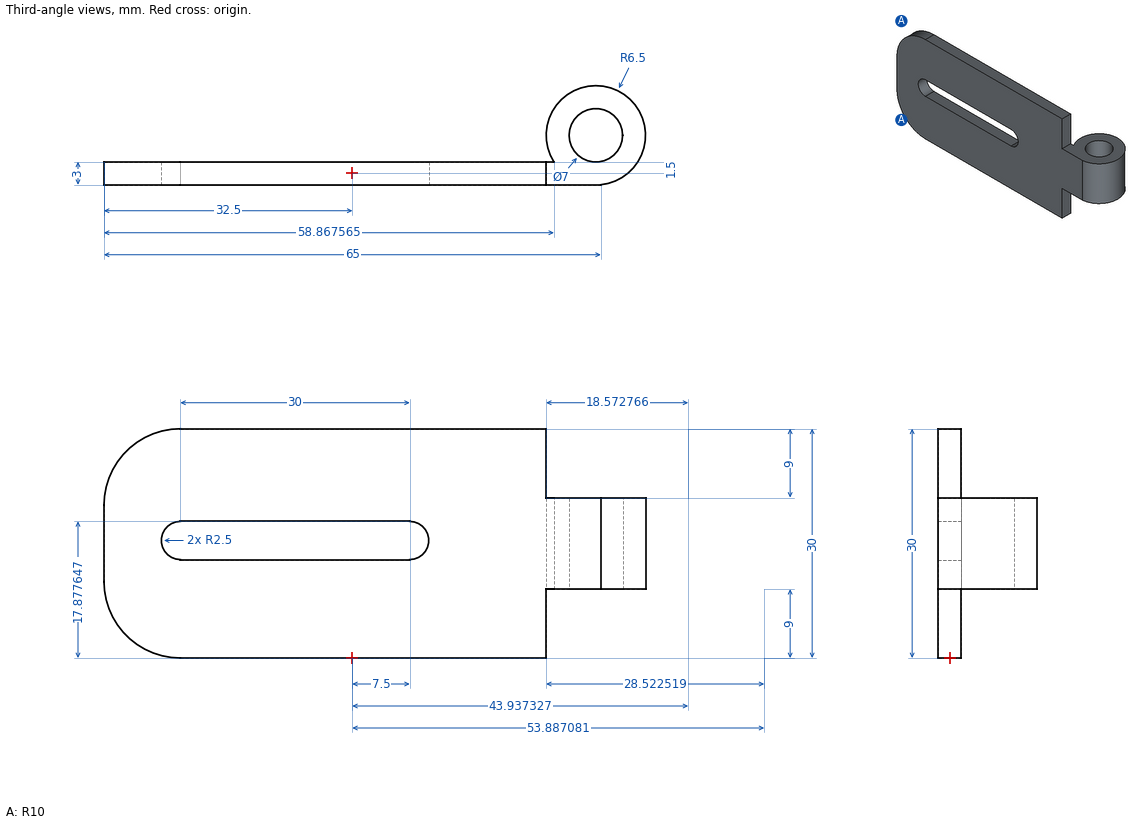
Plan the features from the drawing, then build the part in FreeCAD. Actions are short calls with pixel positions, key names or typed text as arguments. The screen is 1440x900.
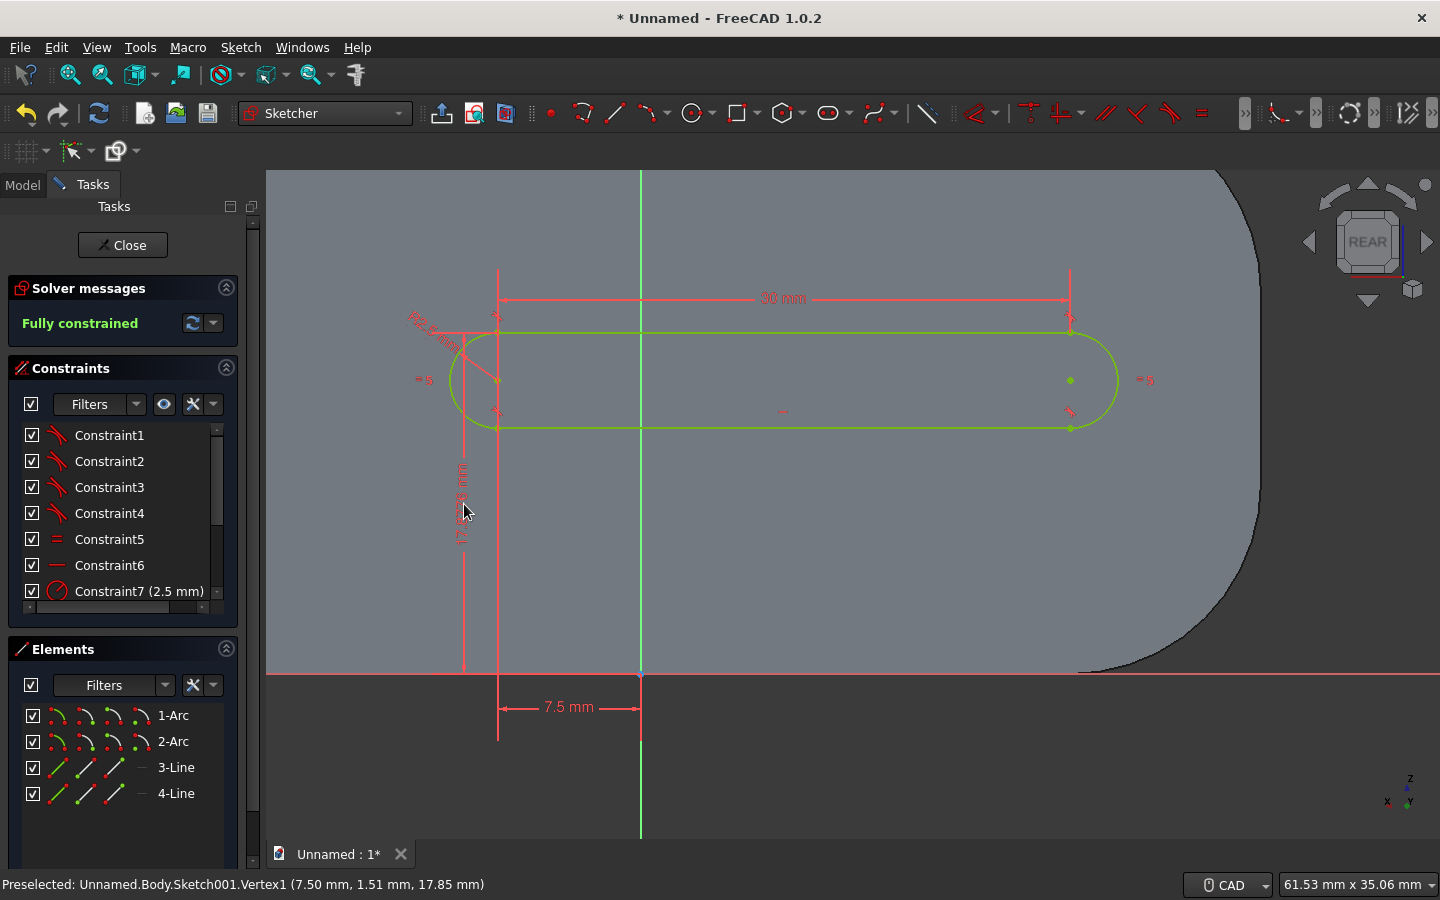
click(123, 245)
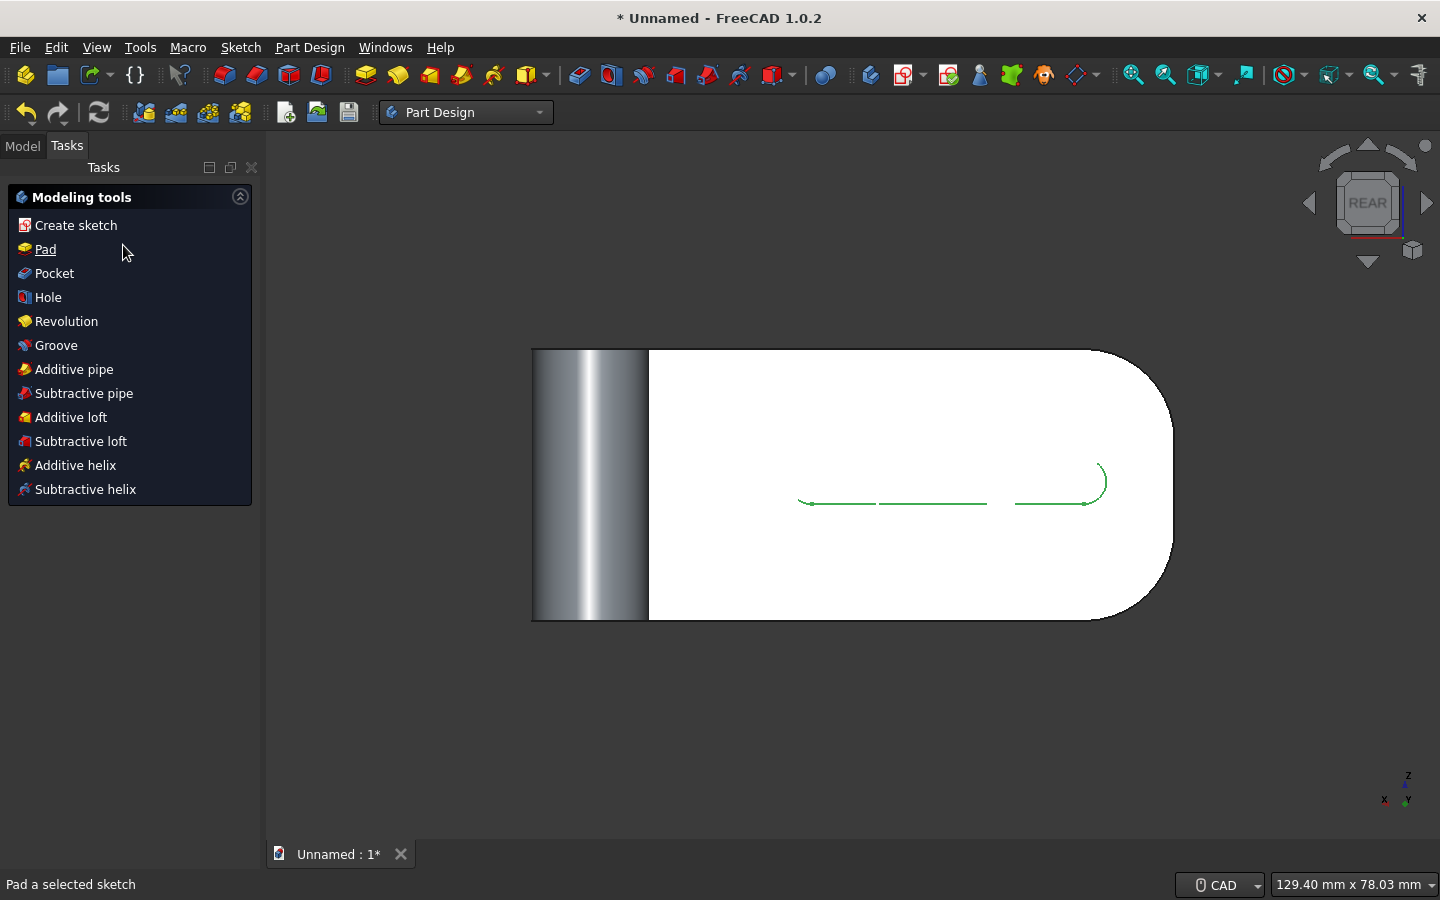
click(580, 76)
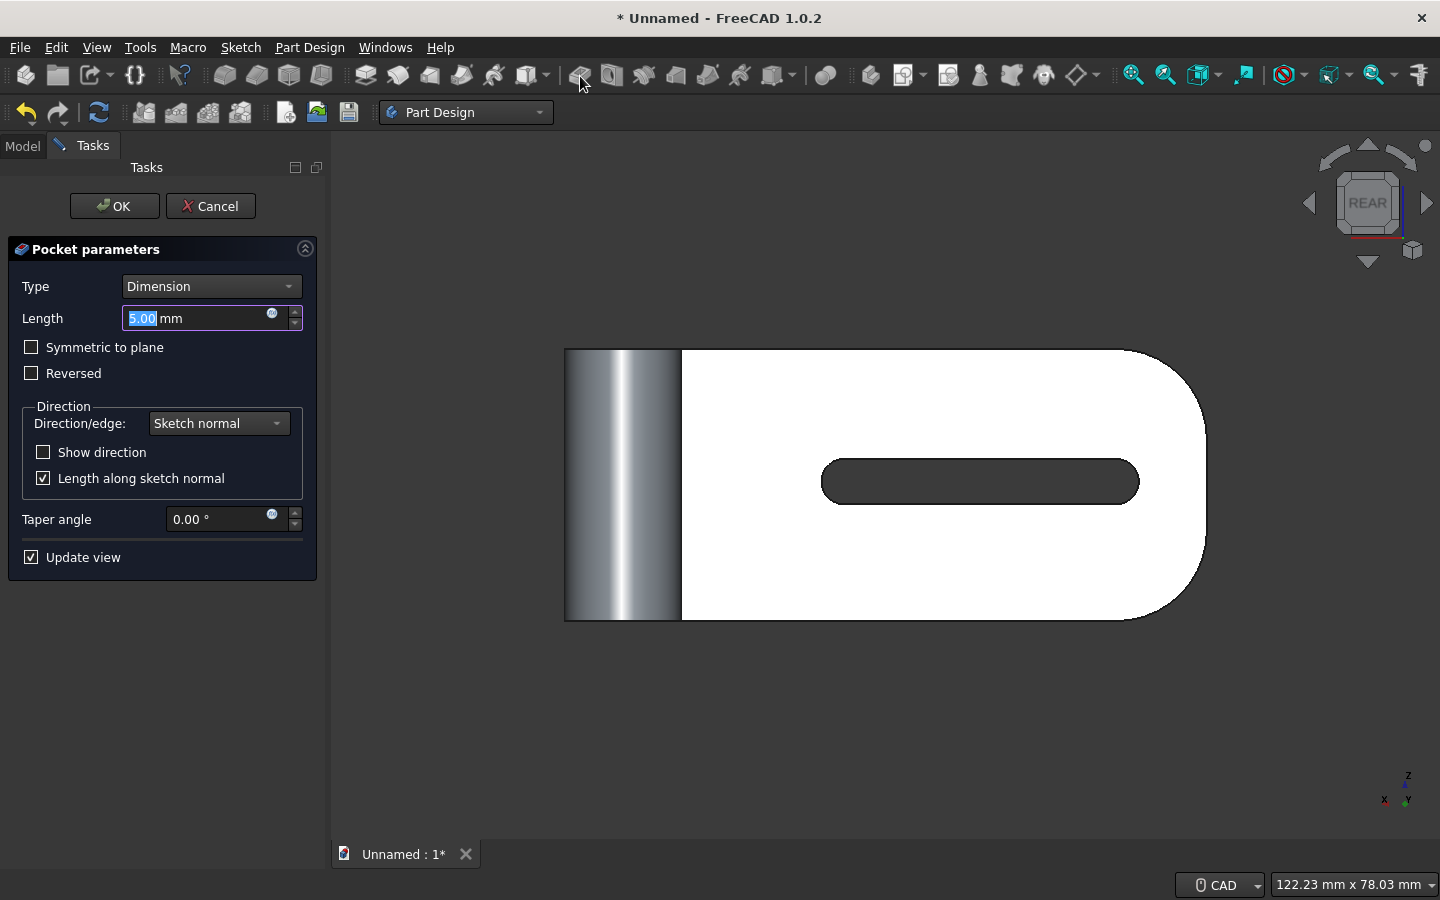
text(30)
key(Tab)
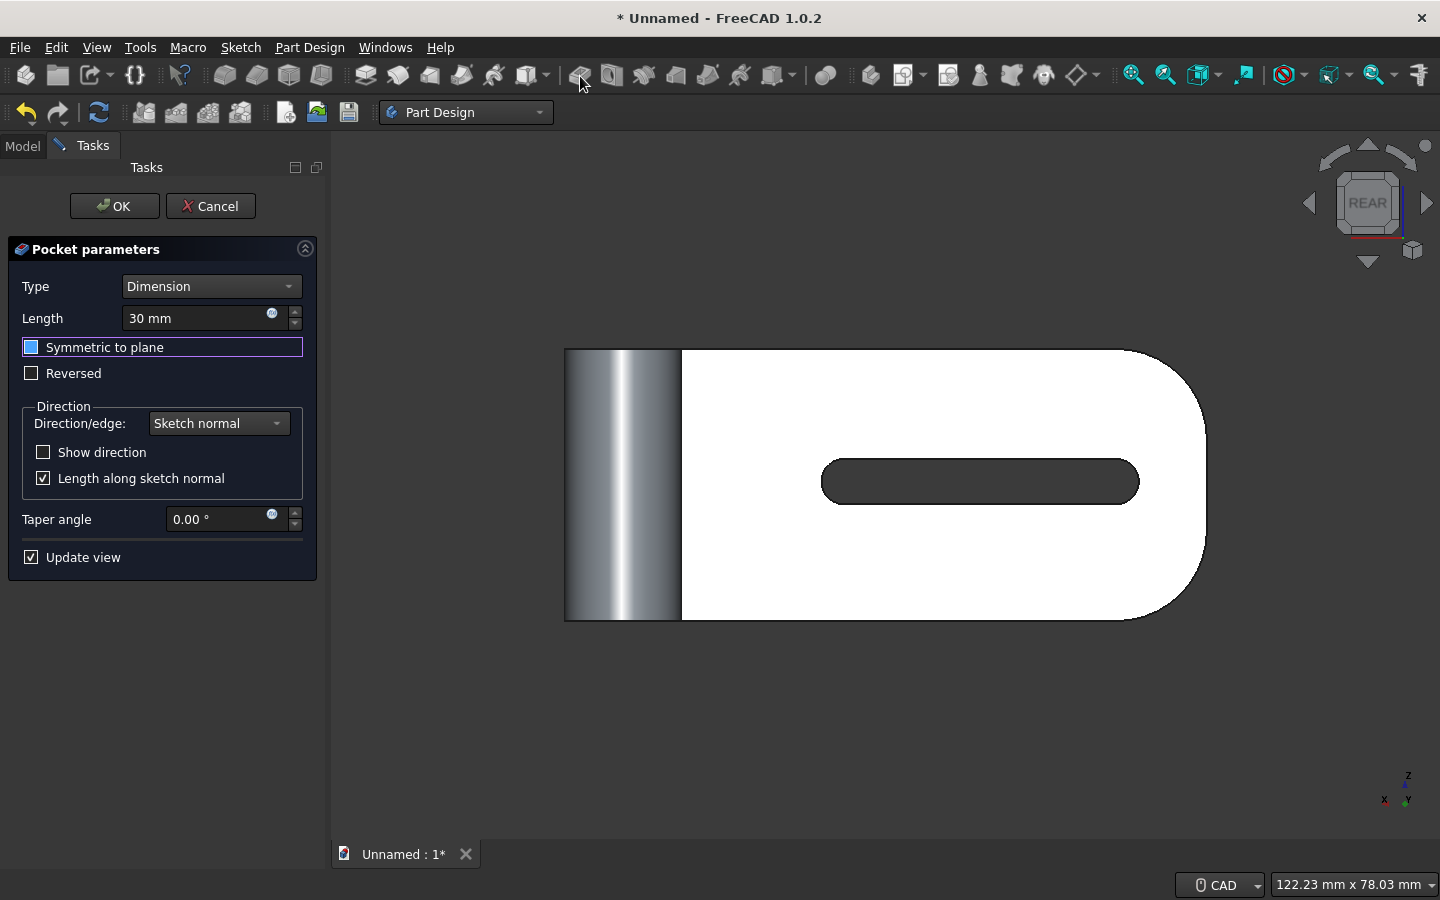
click(115, 206)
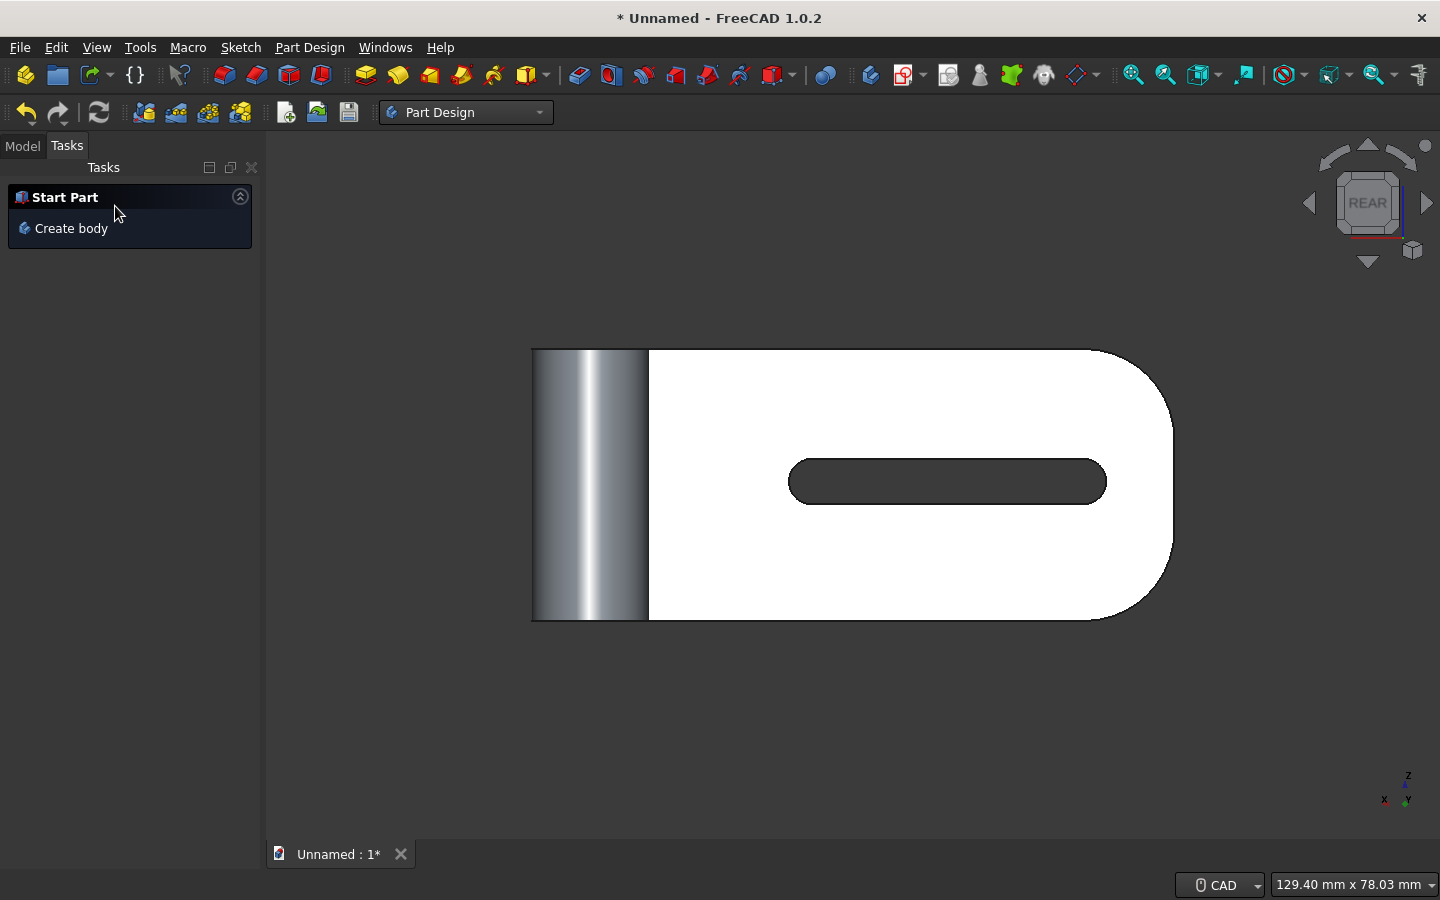
click(755, 406)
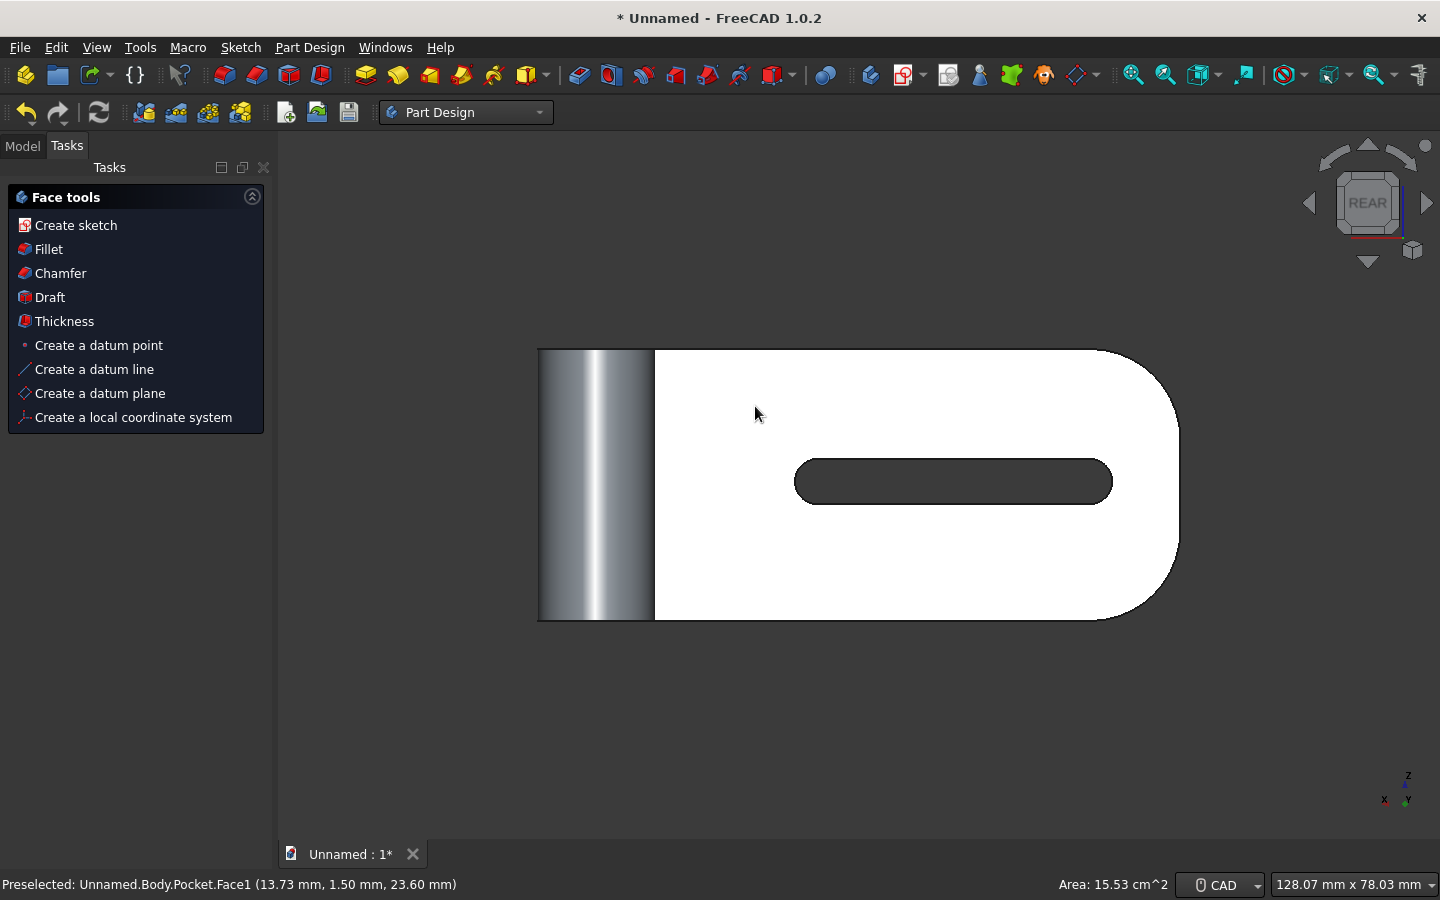
click(904, 76)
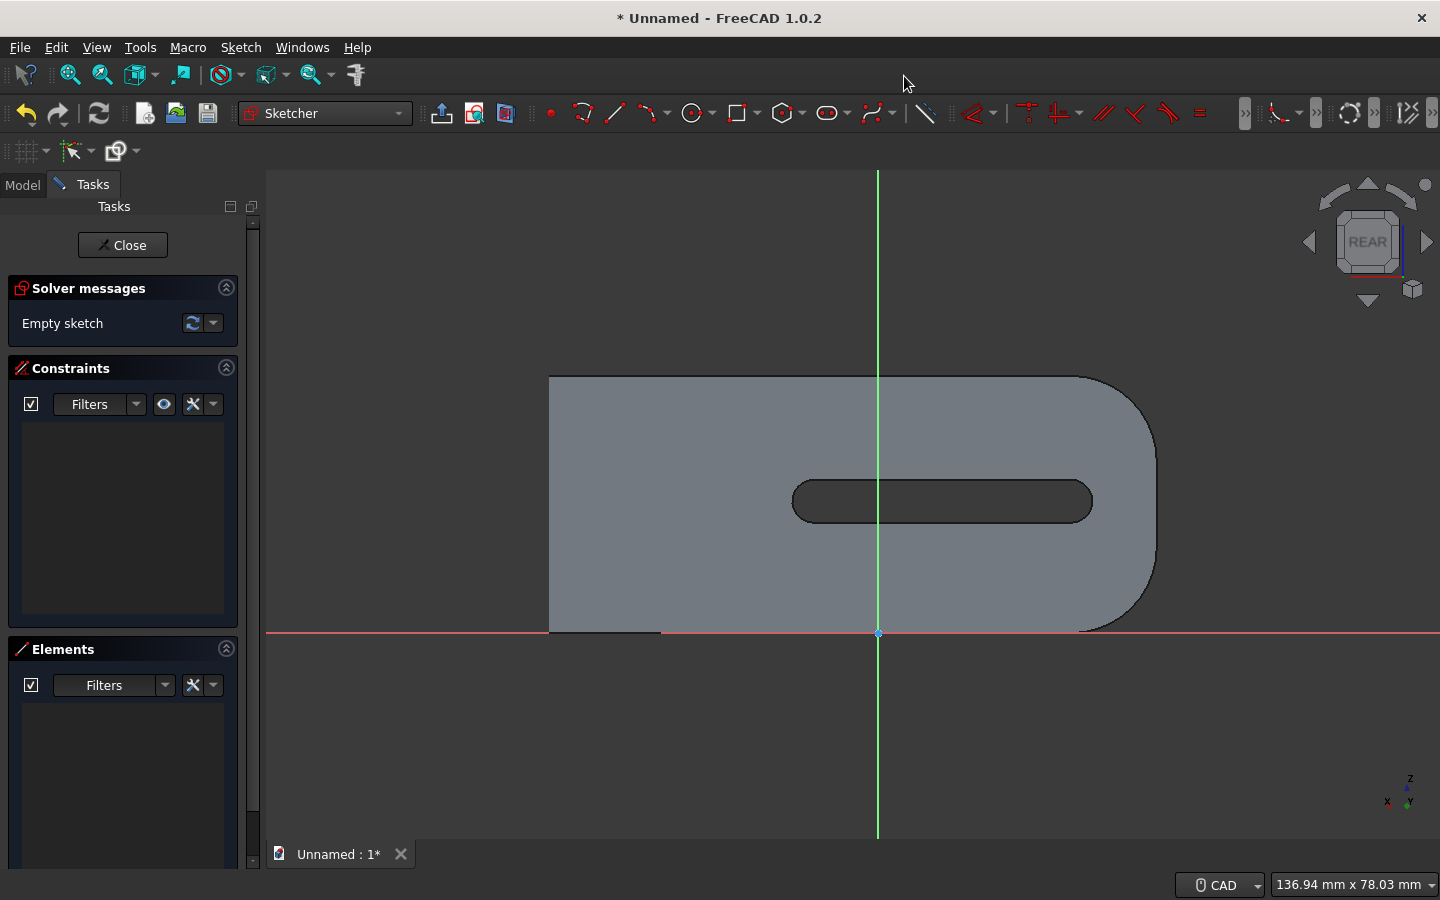
click(506, 114)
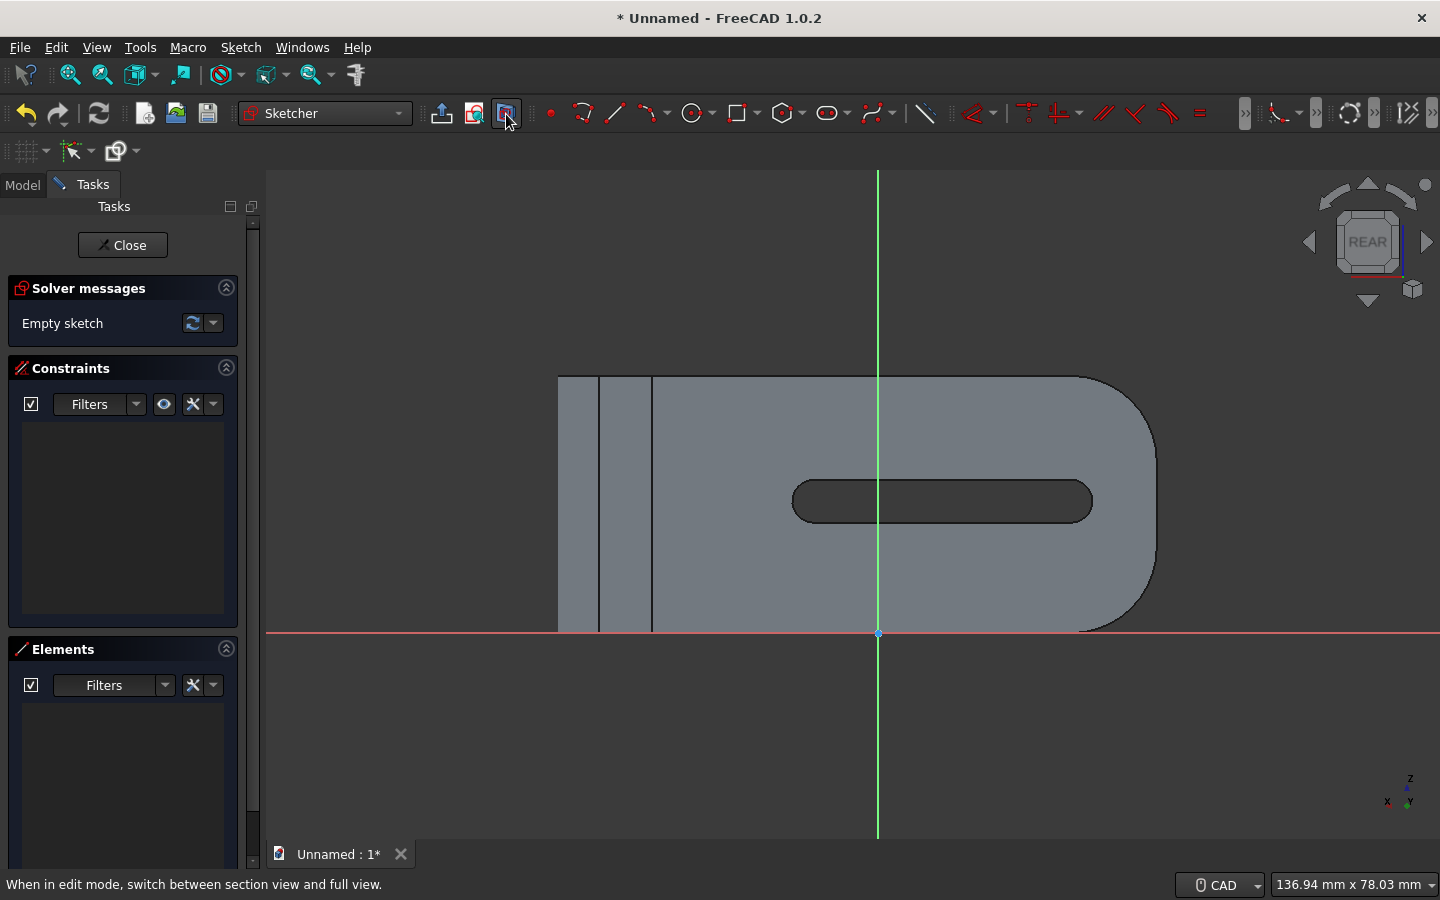
scroll(368, 505, up, 2)